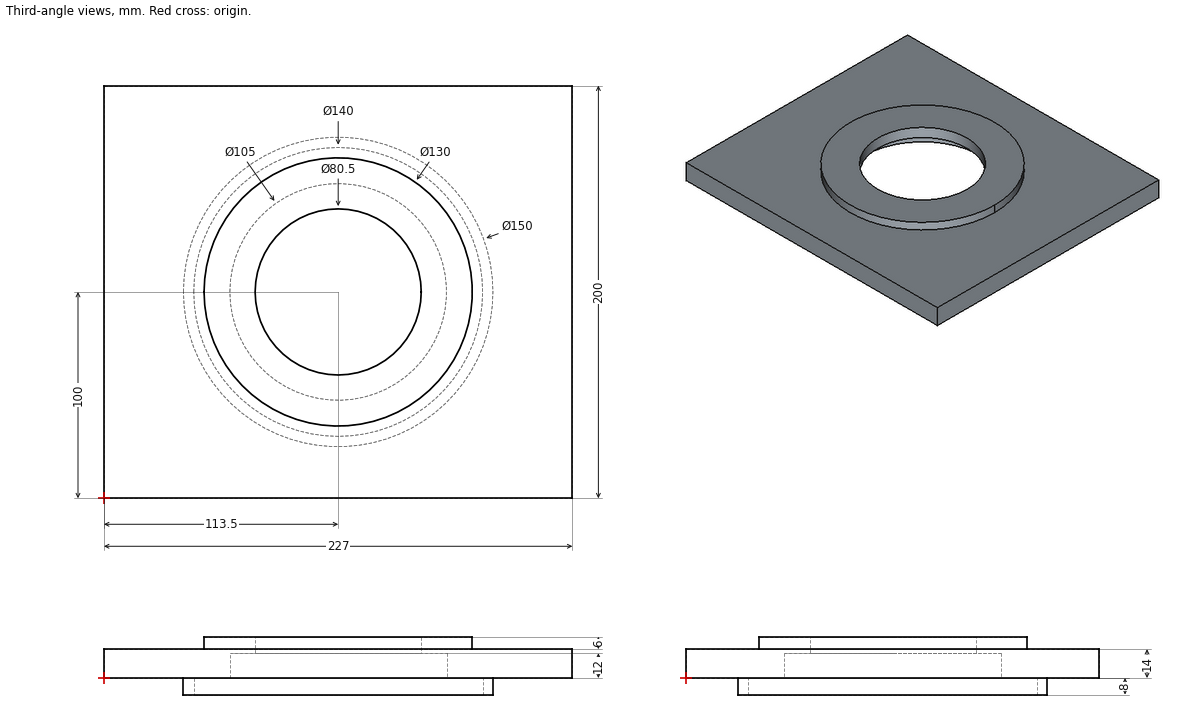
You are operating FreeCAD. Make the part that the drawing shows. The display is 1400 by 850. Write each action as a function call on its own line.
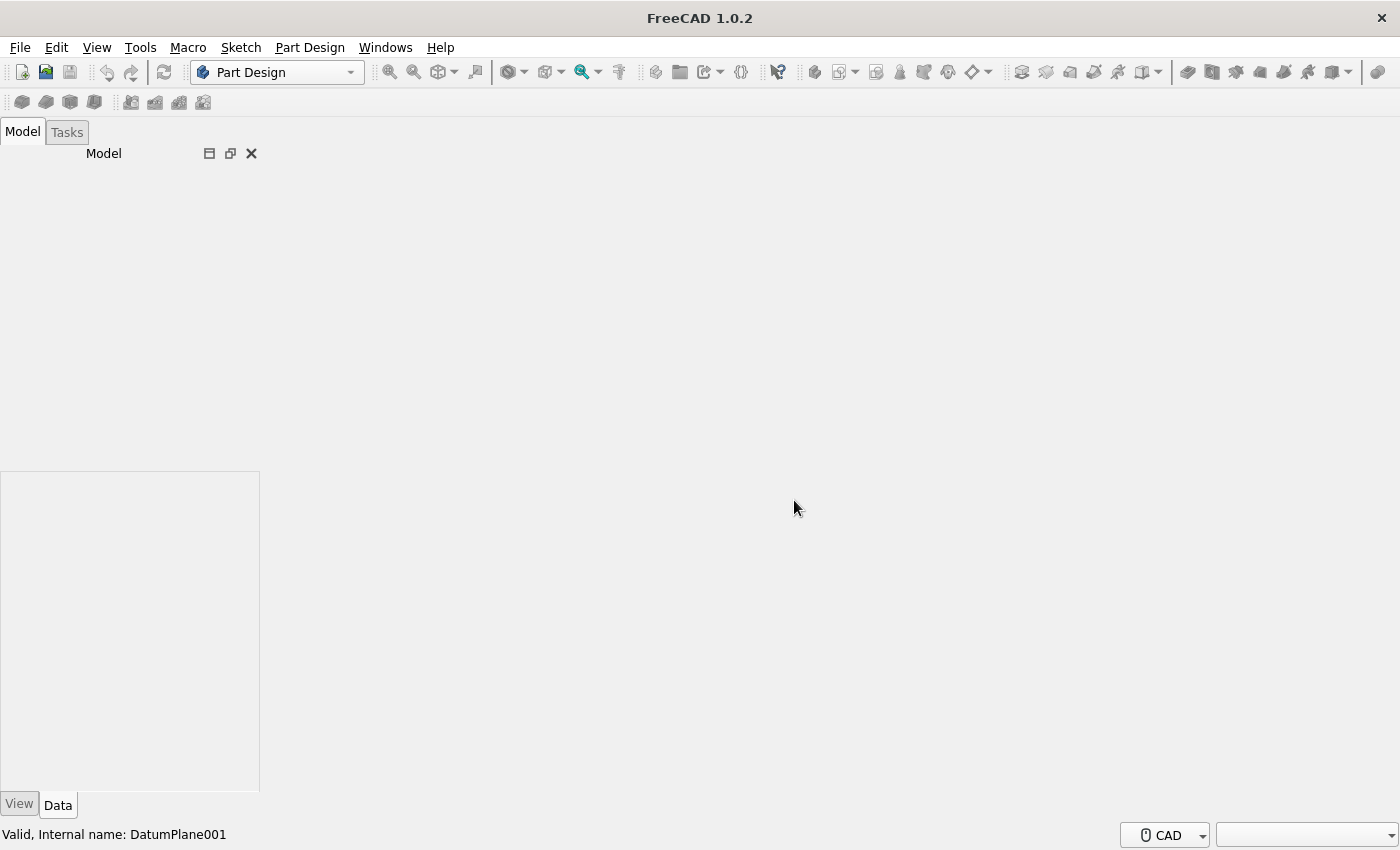
click(22, 72)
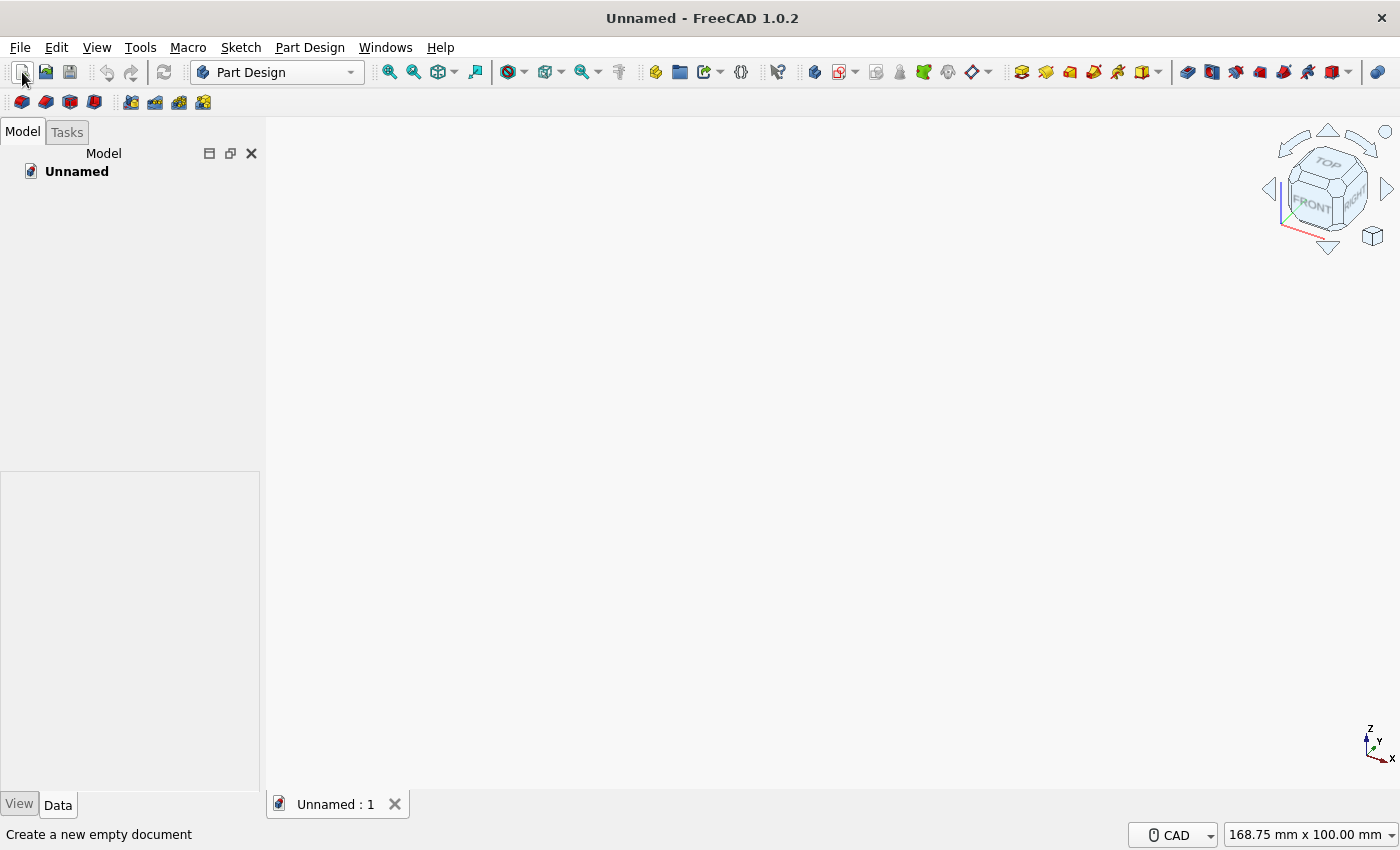
click(840, 72)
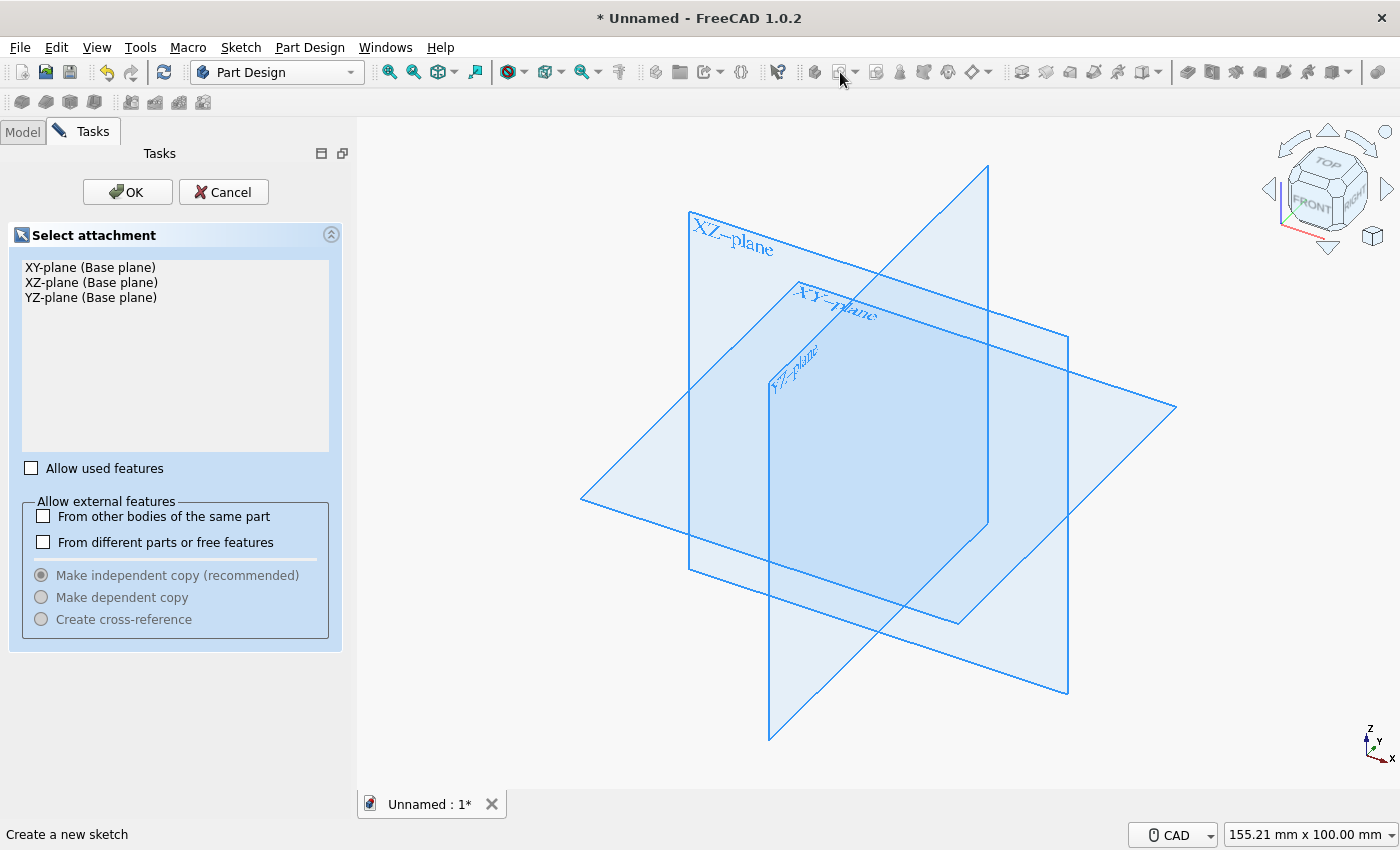
click(82, 268)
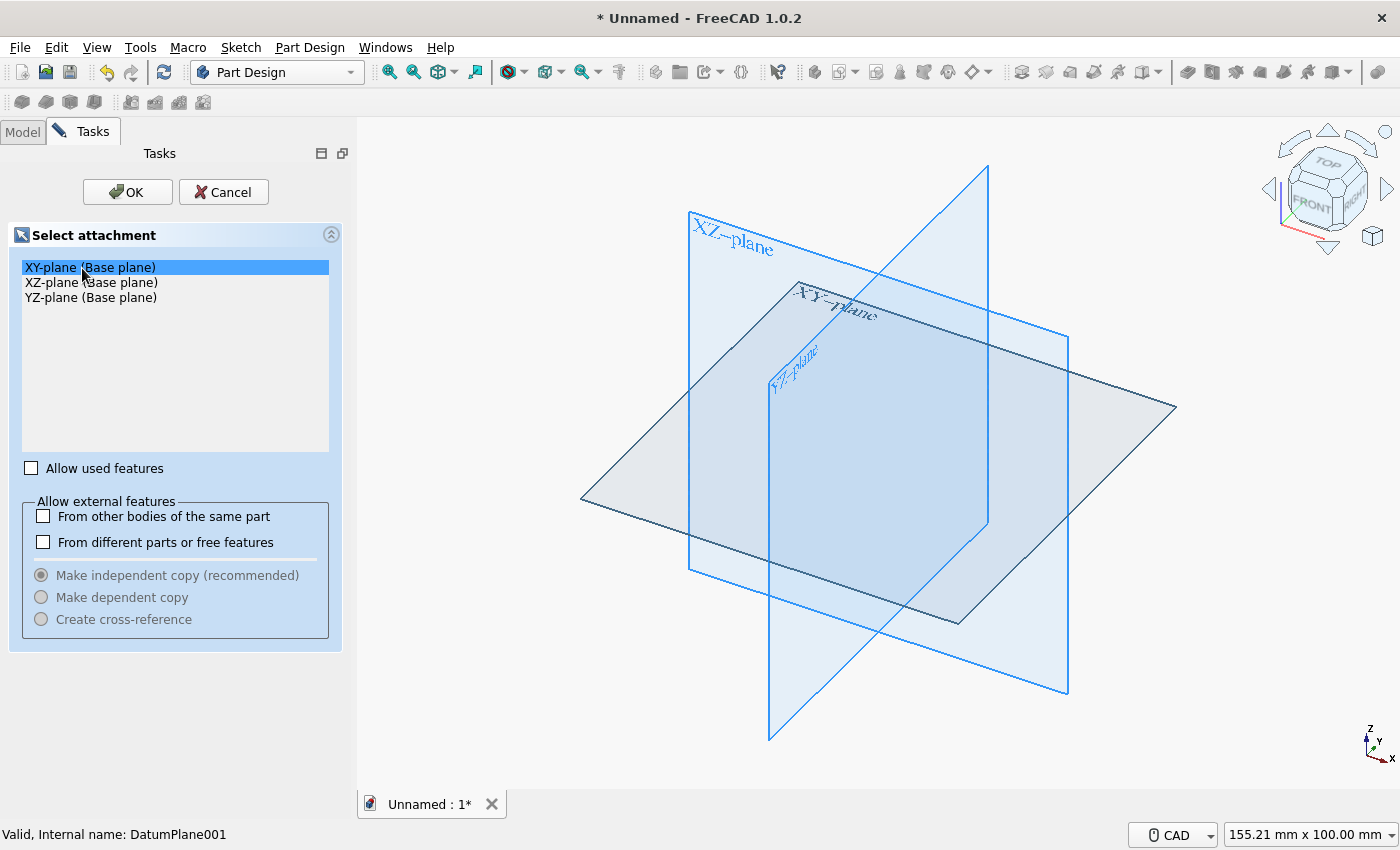
click(128, 192)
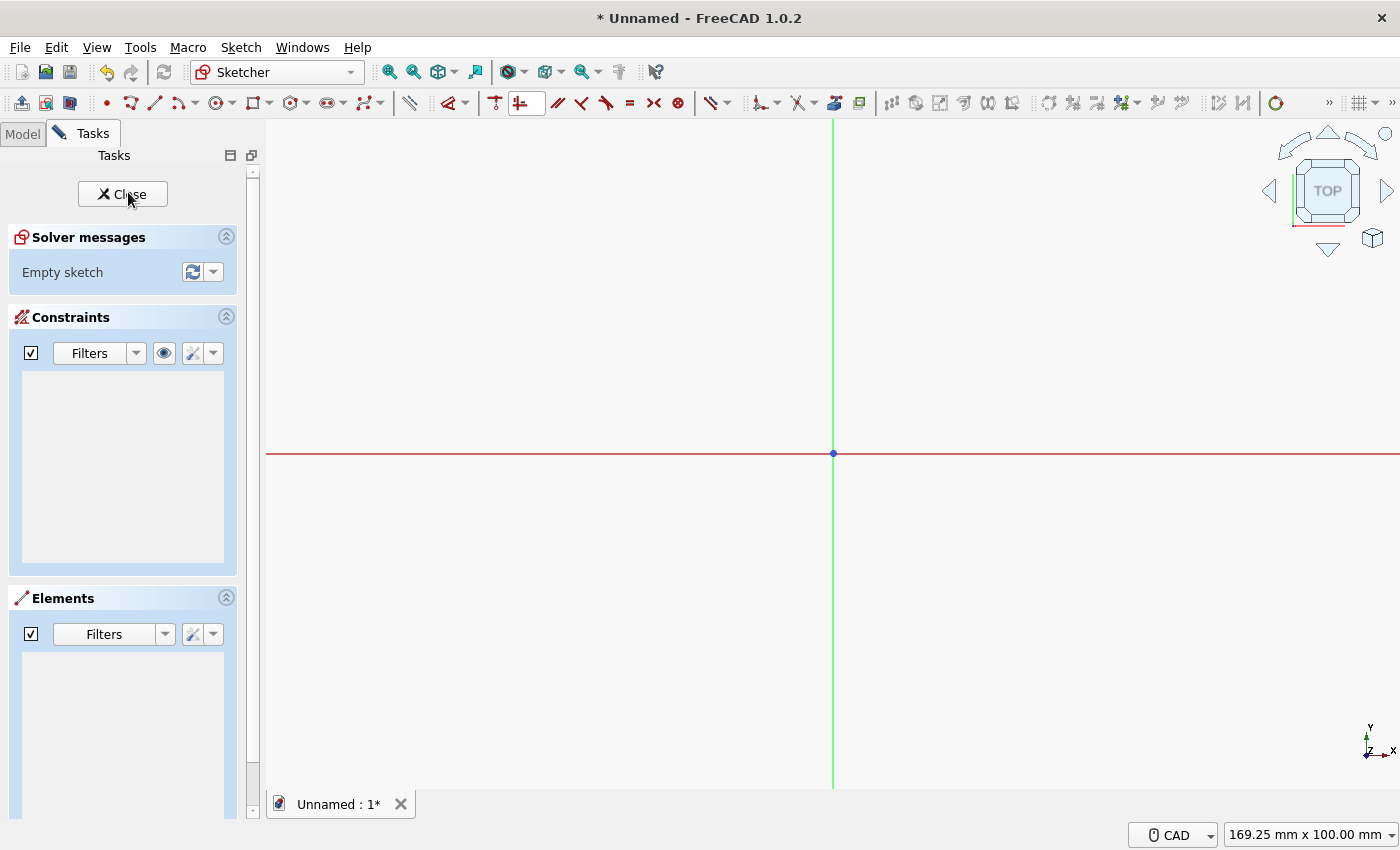
scroll(407, 743, down, 6)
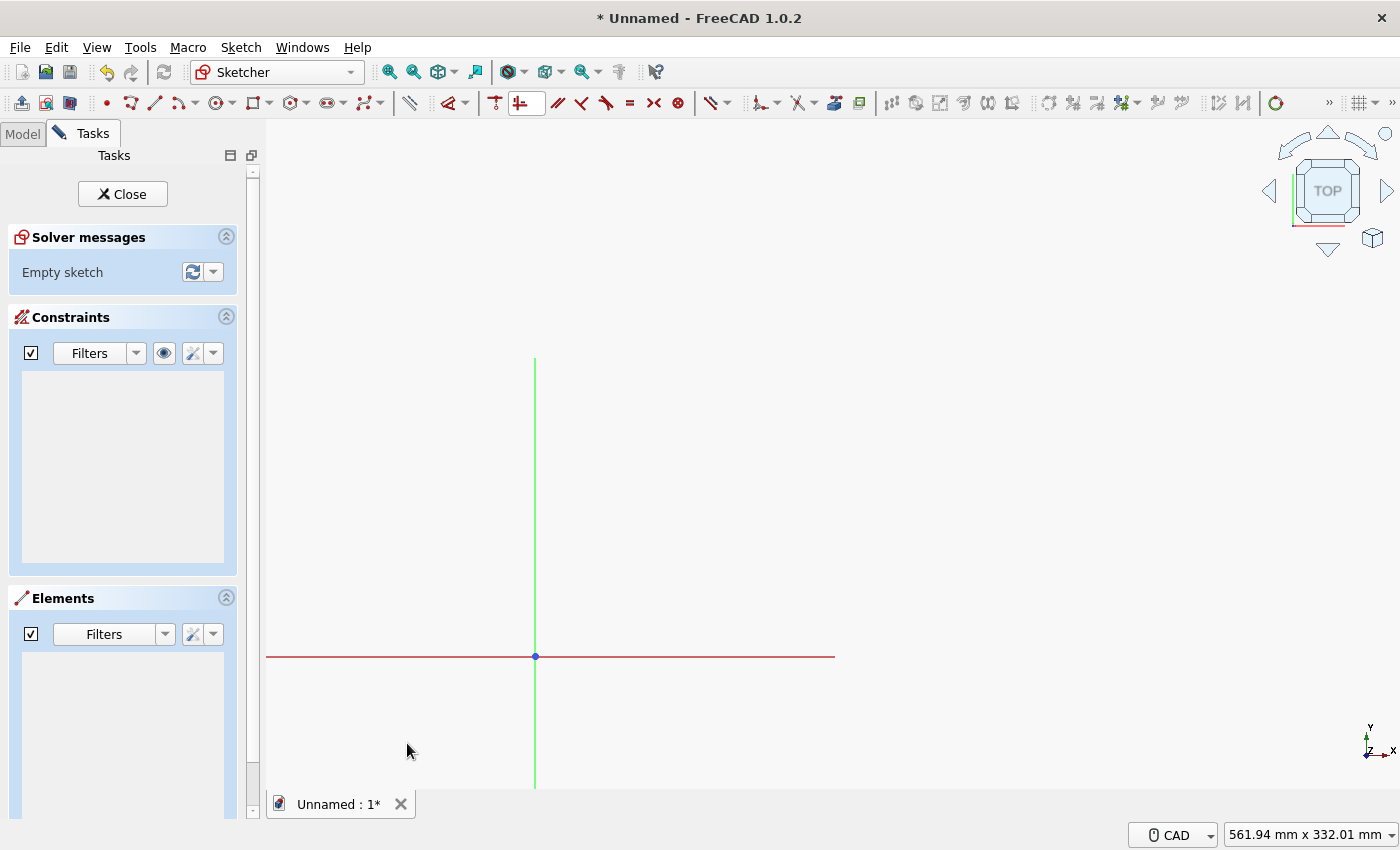
key(g)
key(r)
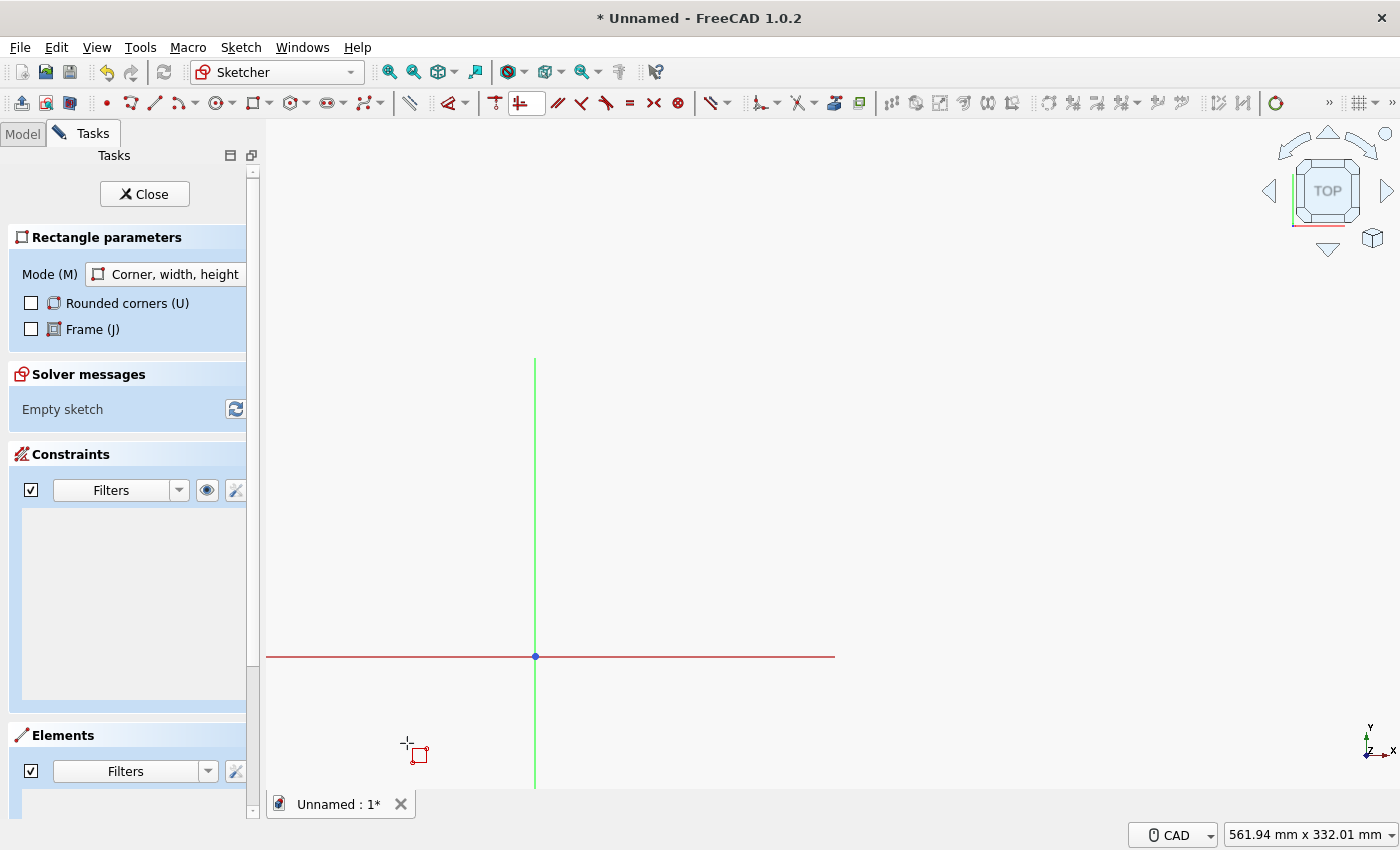
click(535, 657)
click(993, 253)
key(Escape)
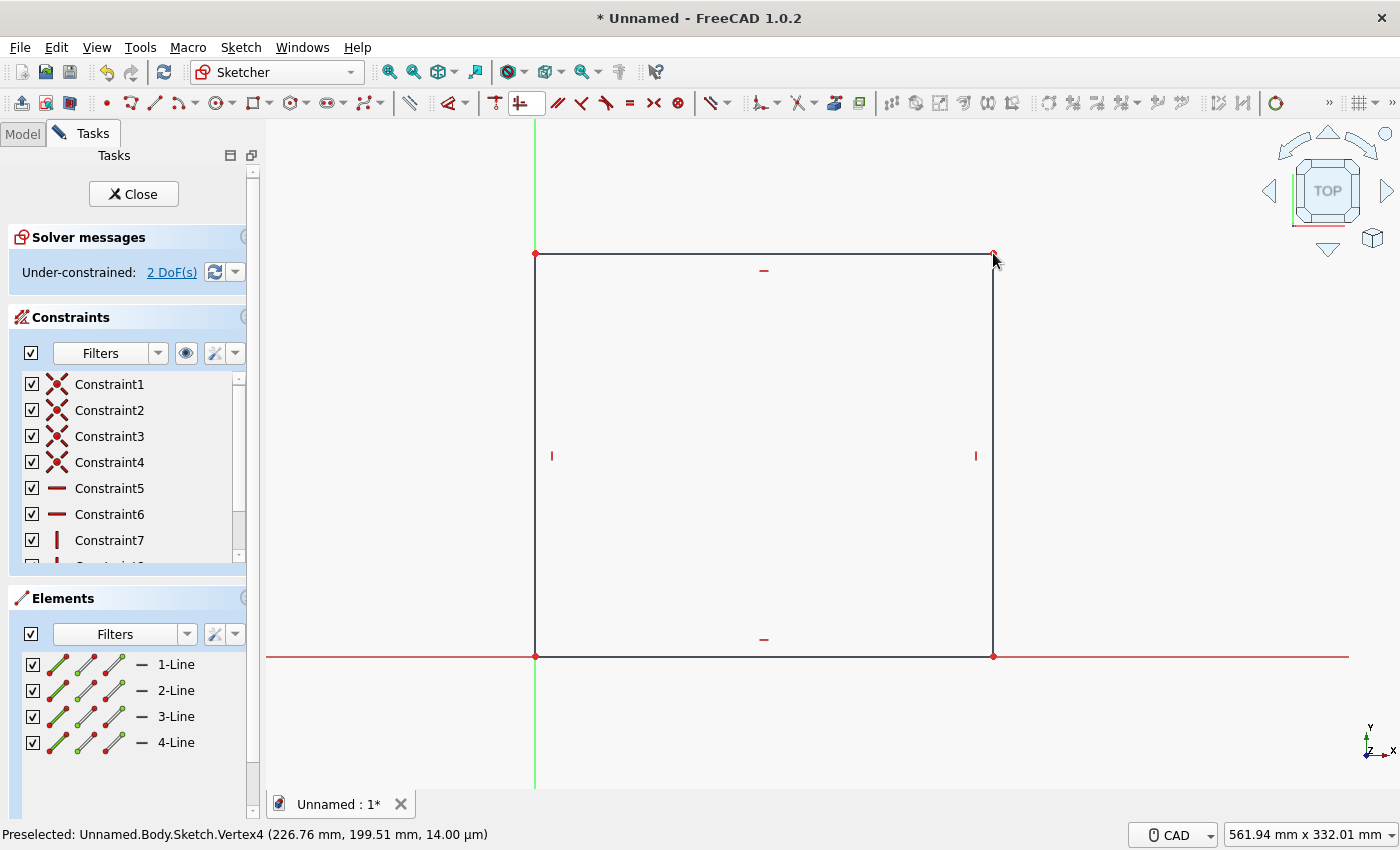
key(d)